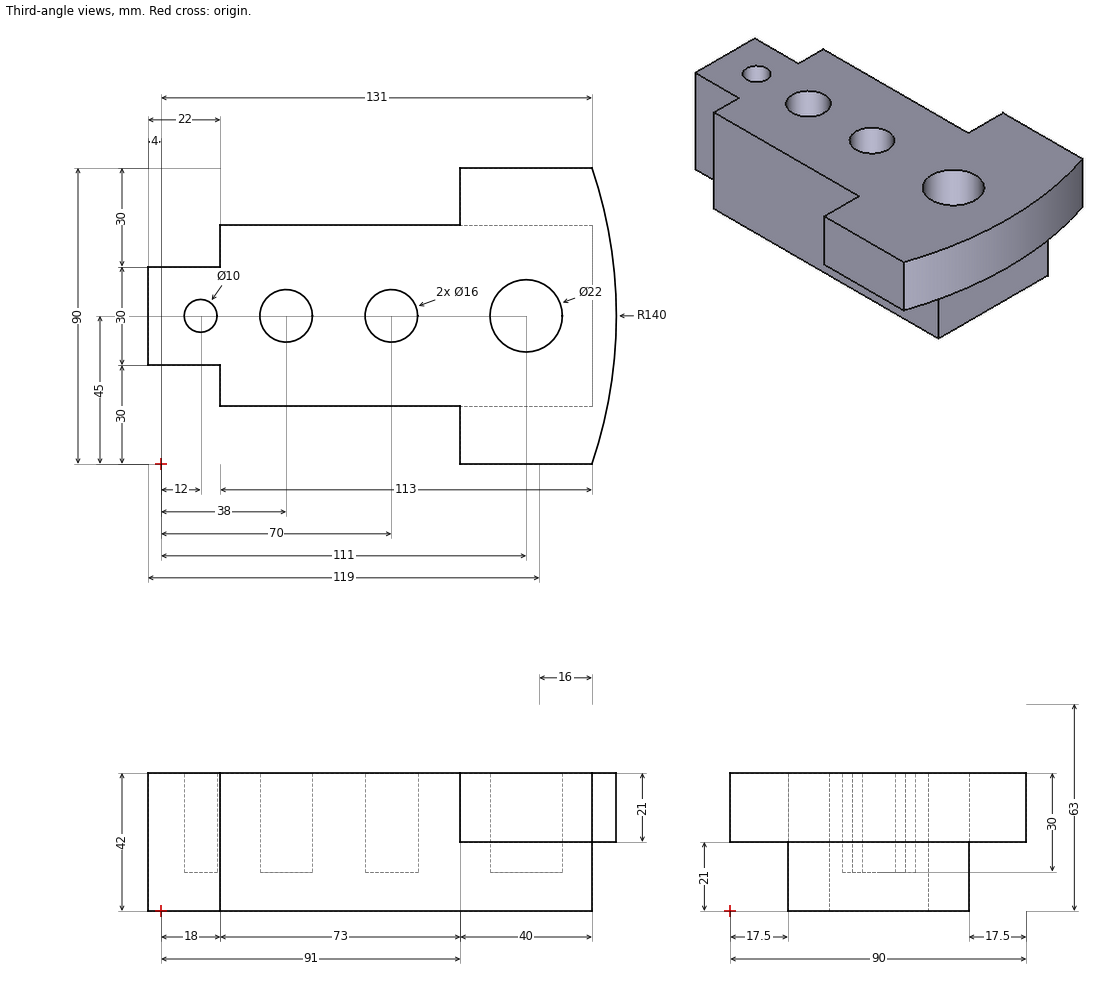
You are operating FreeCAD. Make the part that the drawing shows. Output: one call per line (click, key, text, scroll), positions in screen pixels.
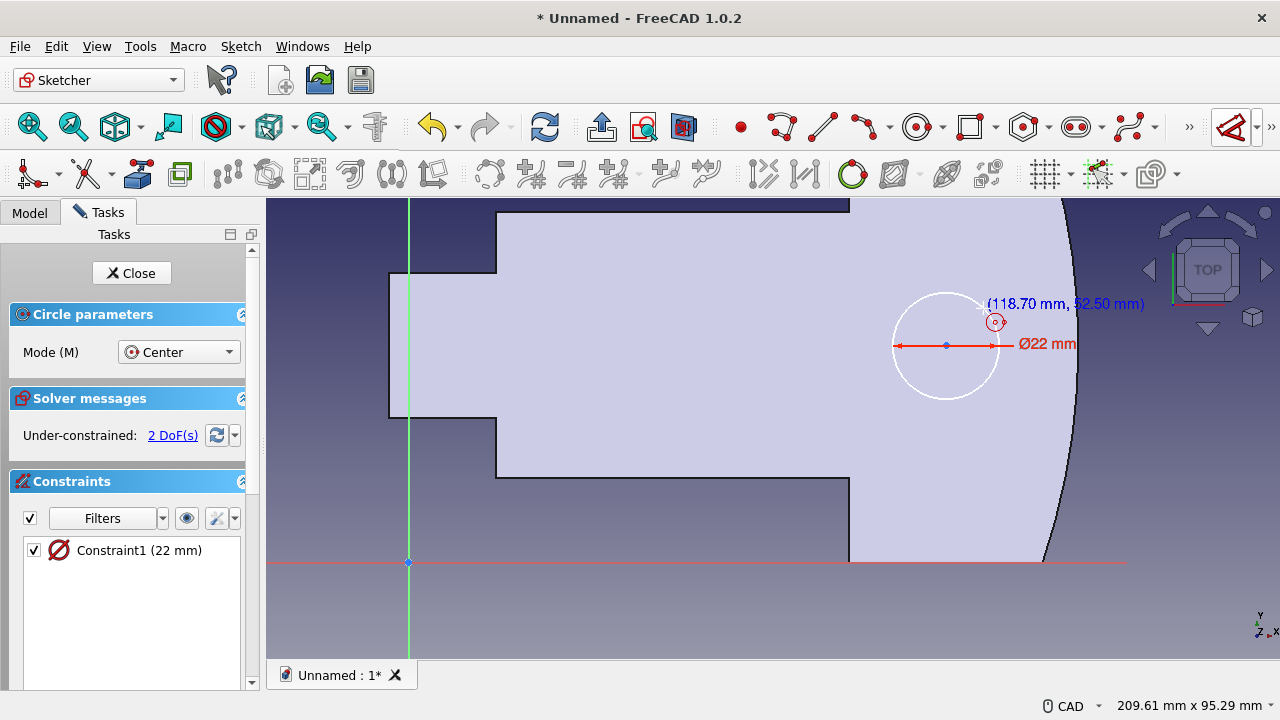
click(747, 345)
move(775, 318)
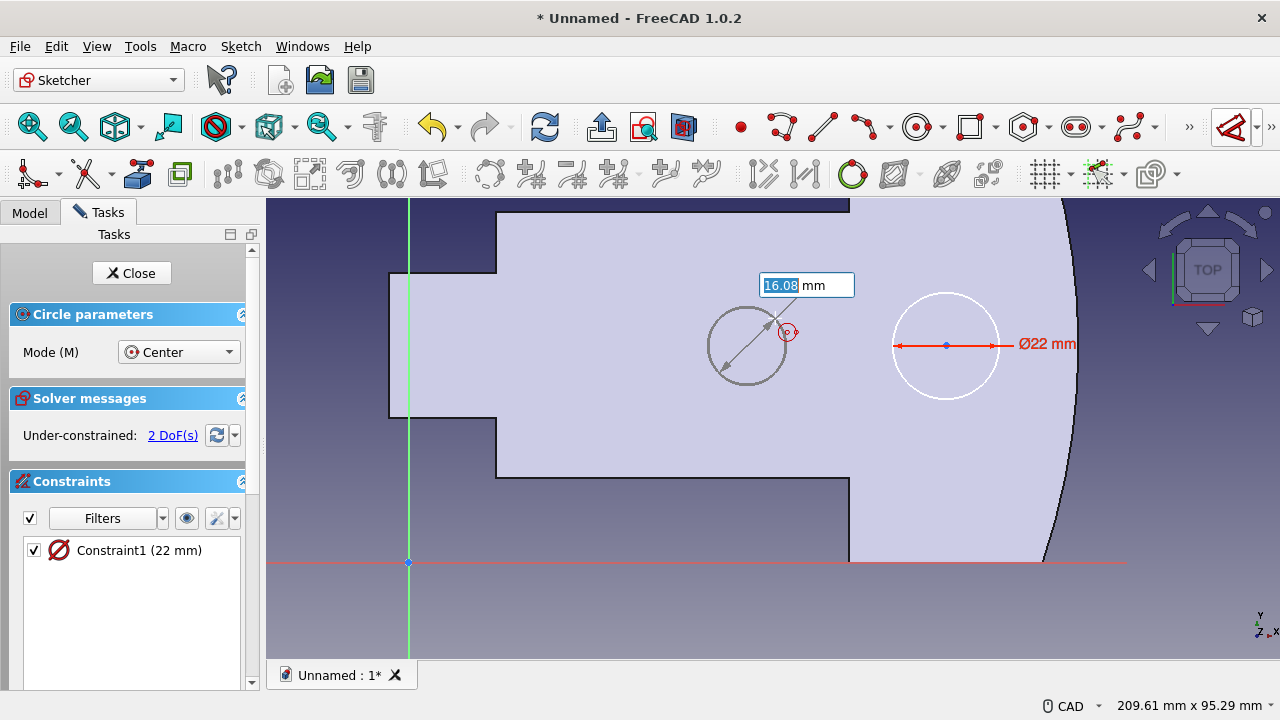
text(16)
key(Return)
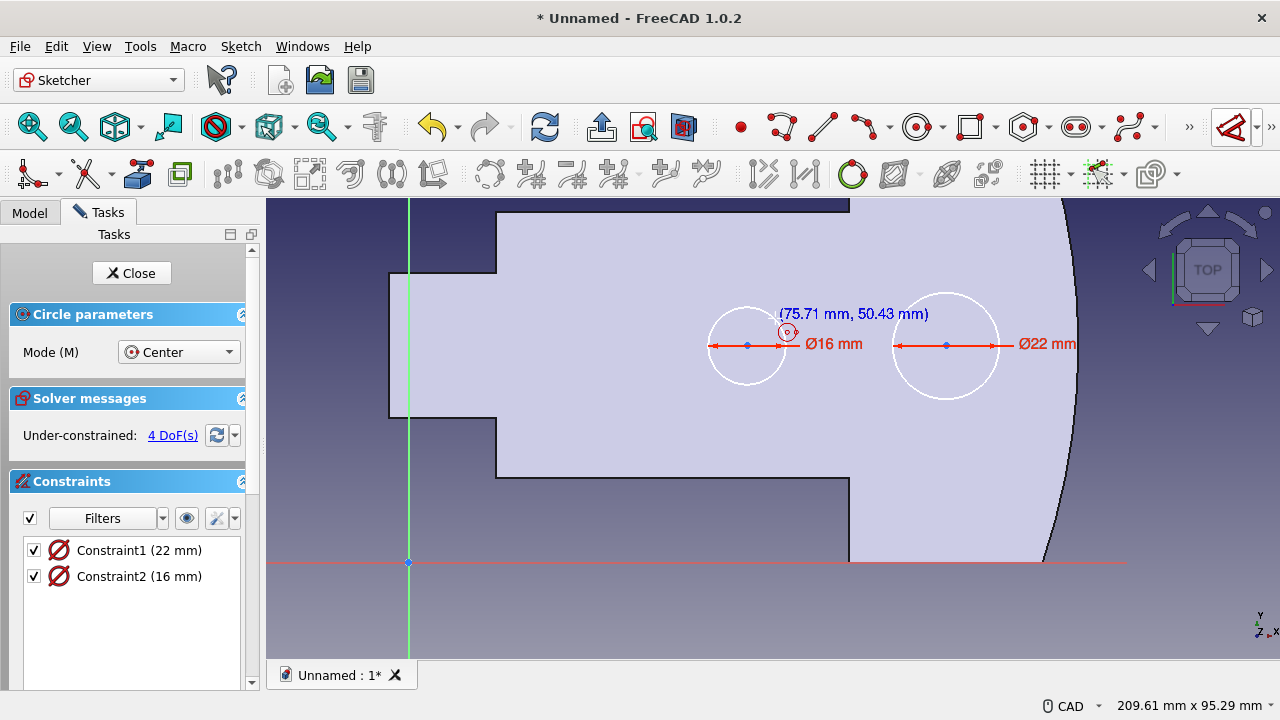
click(593, 345)
move(620, 318)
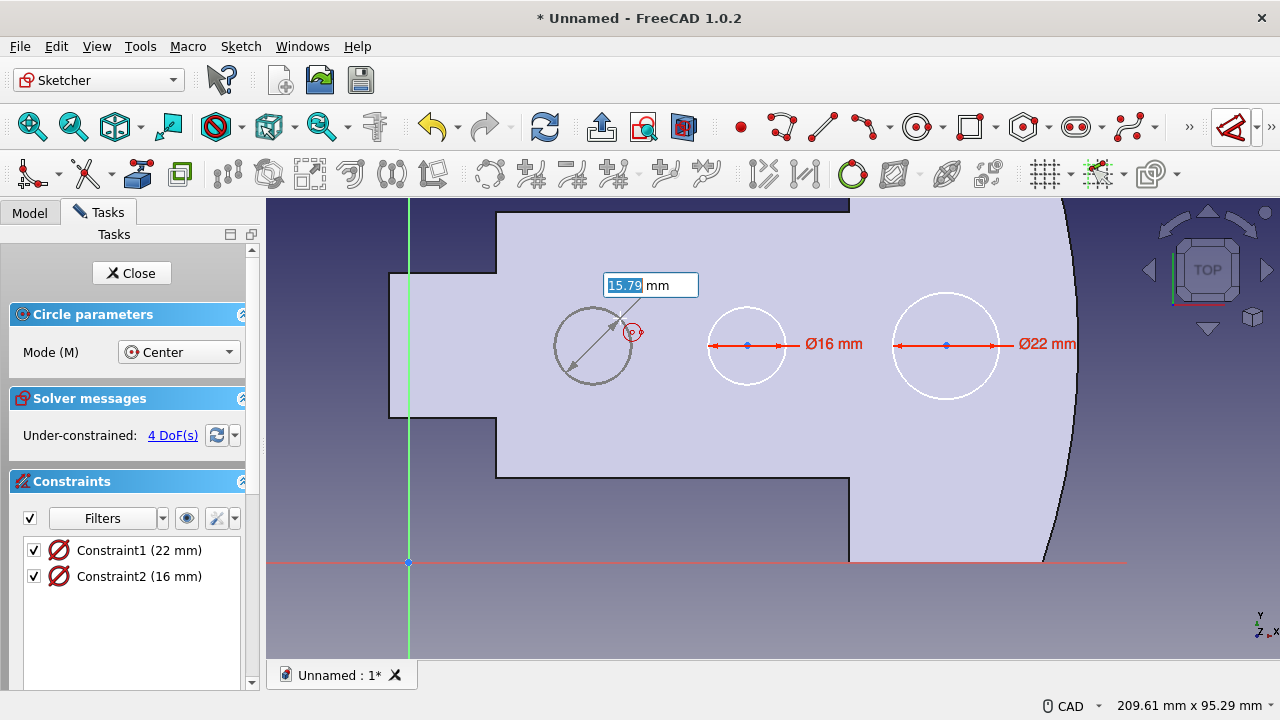
text(16)
key(Return)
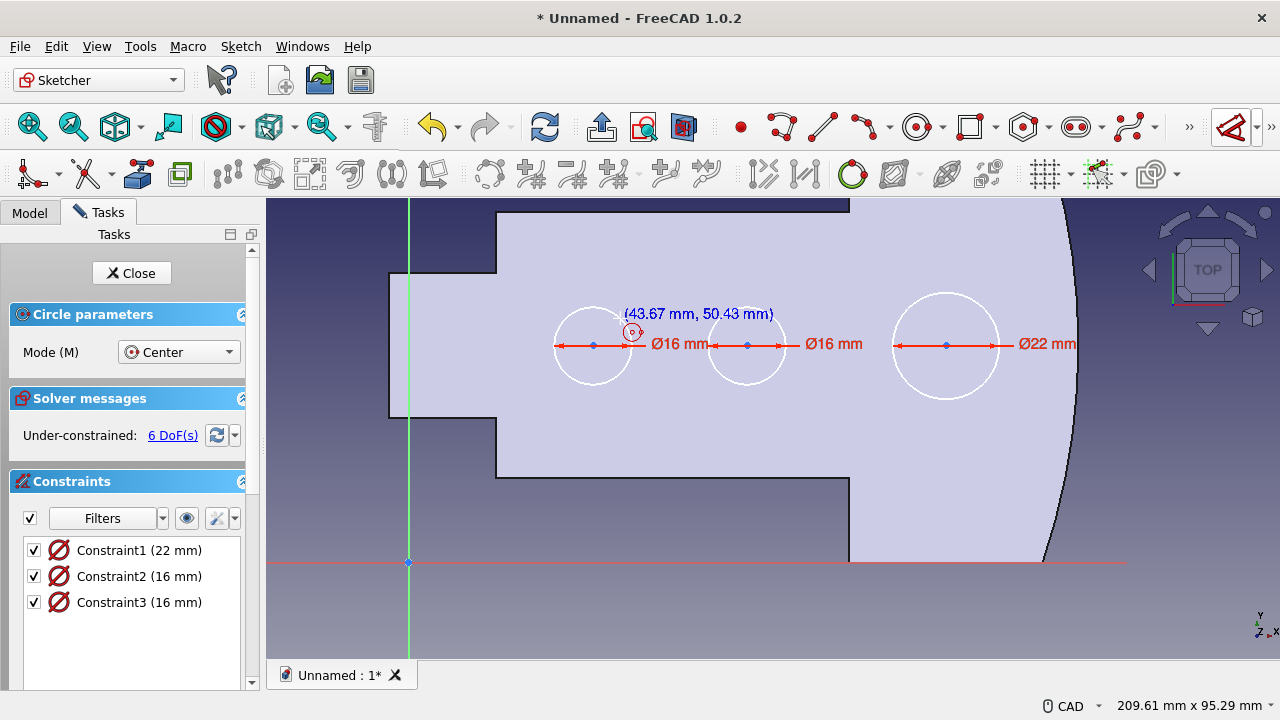
click(467, 345)
move(484, 328)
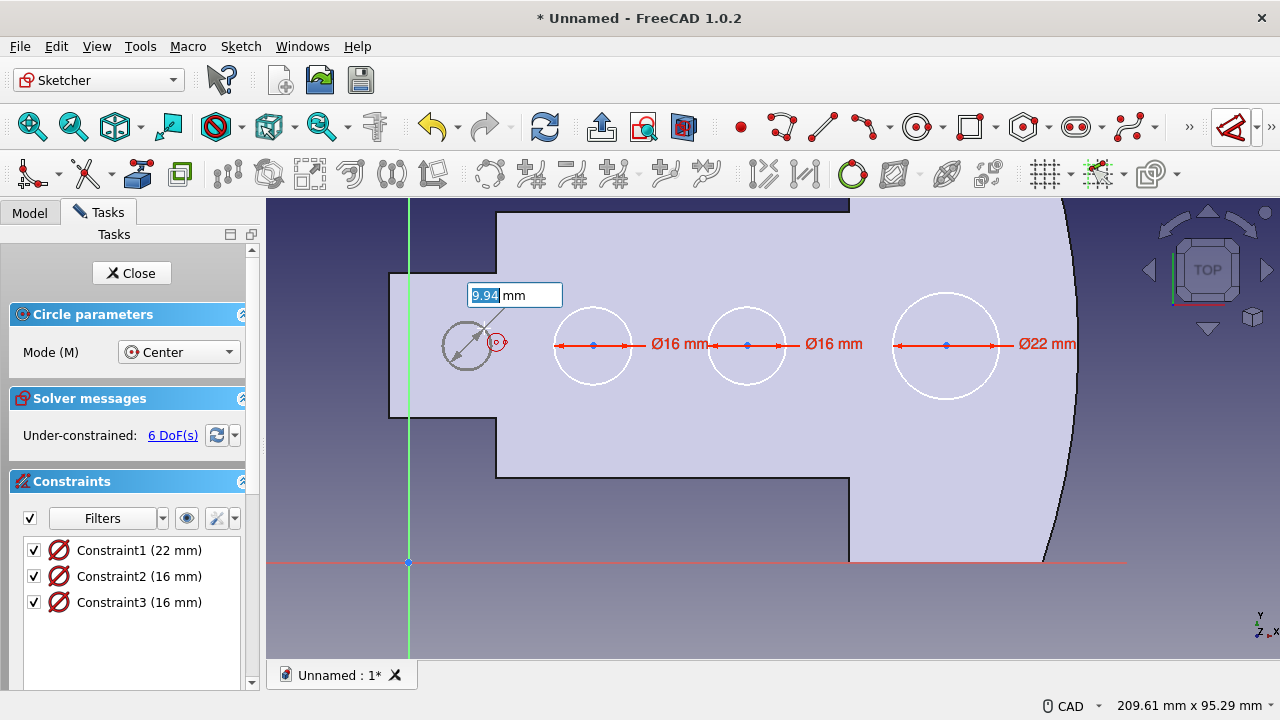
text(10)
key(Return)
key(Escape)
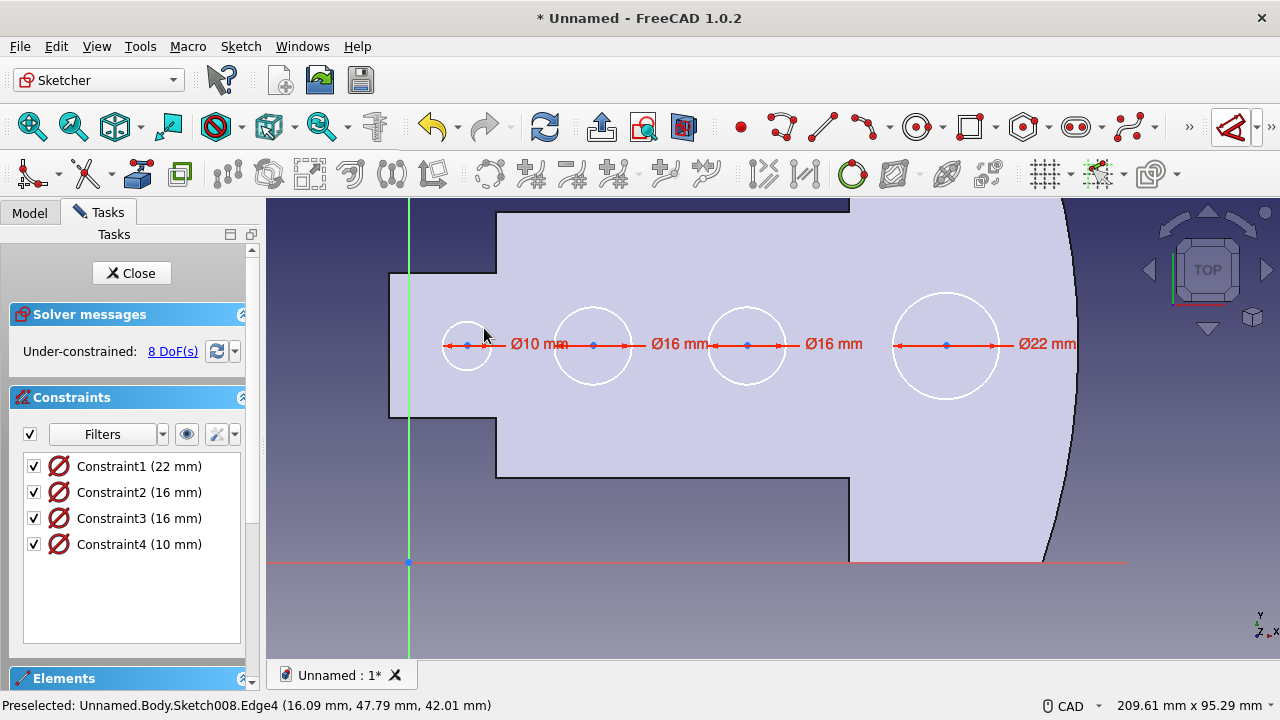
click(946, 346)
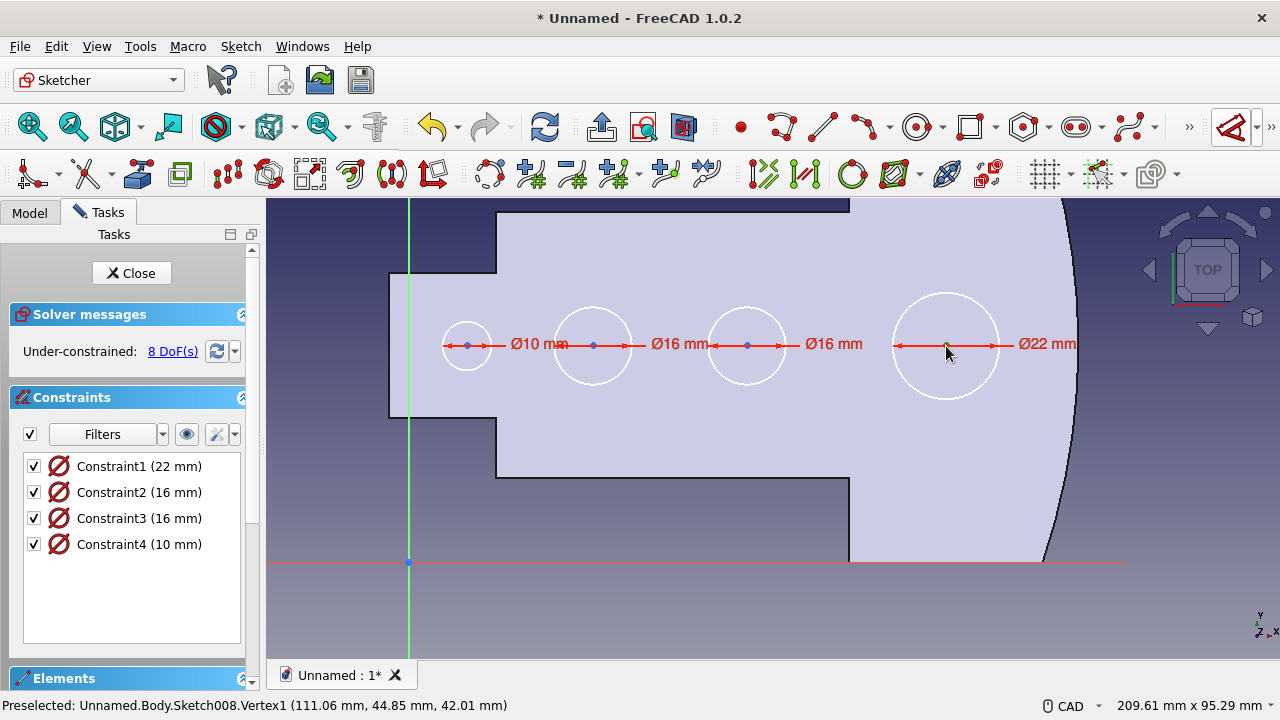
click(747, 346)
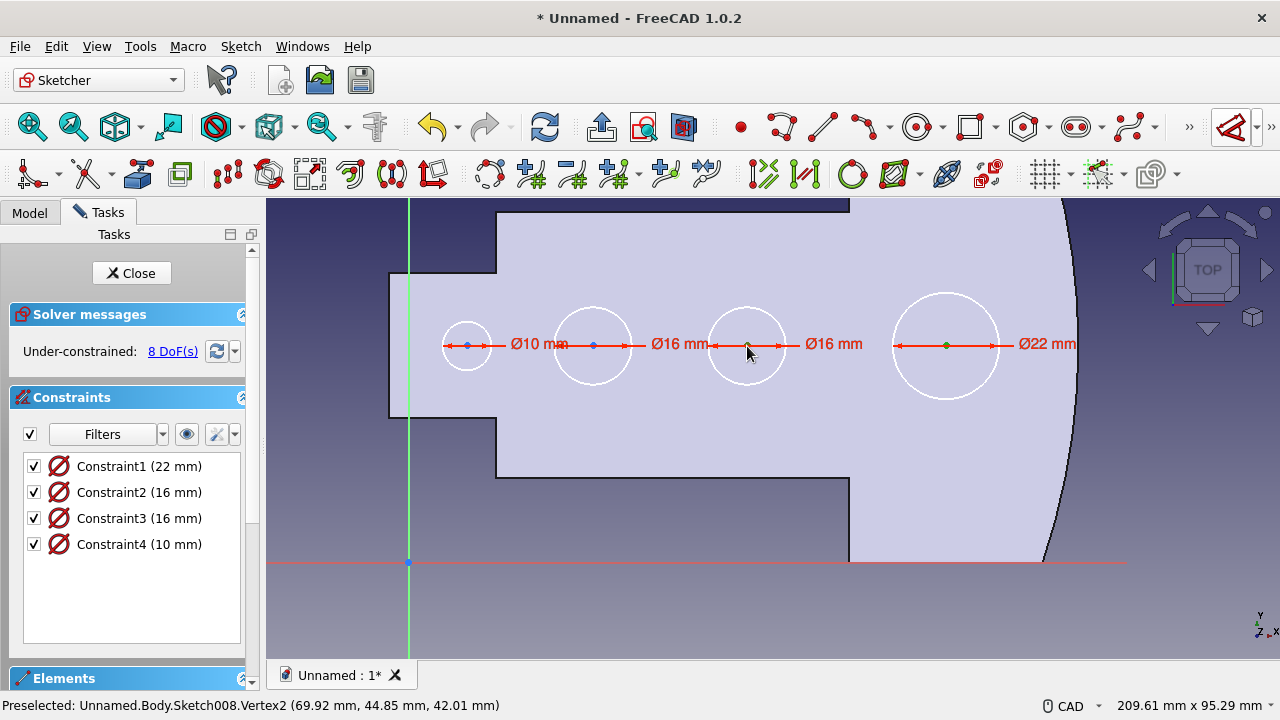
key(h)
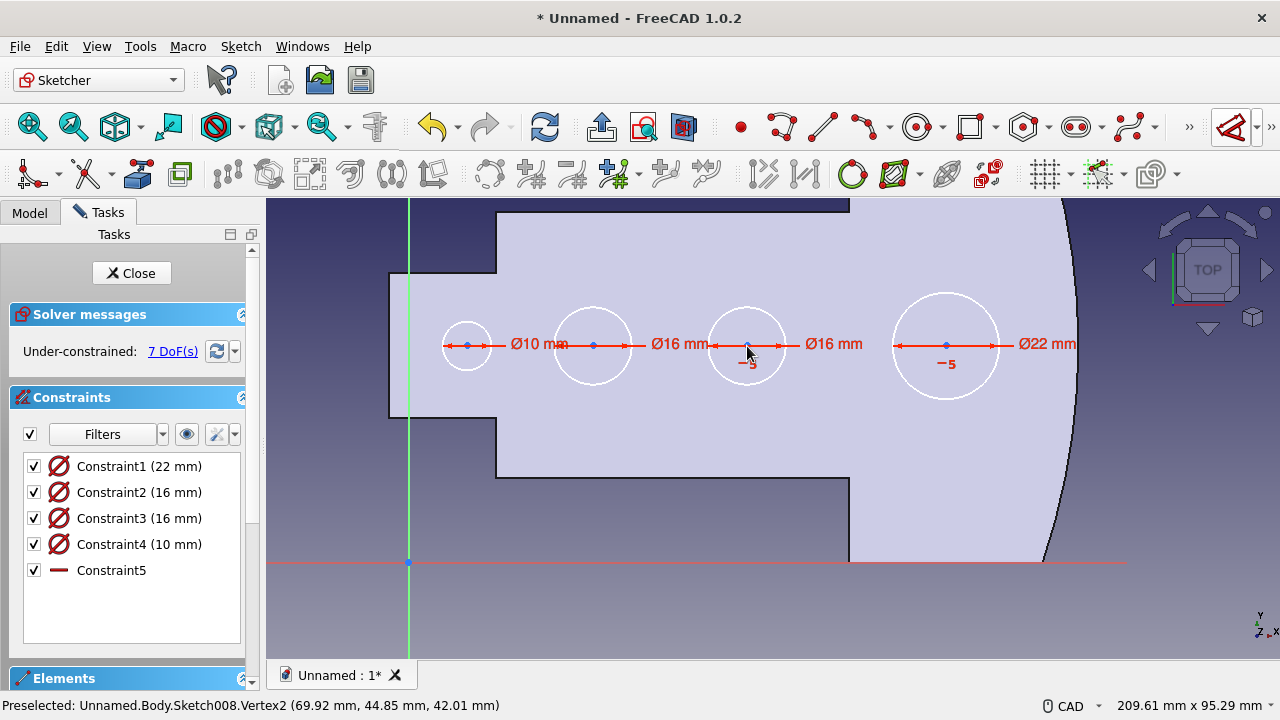
click(747, 346)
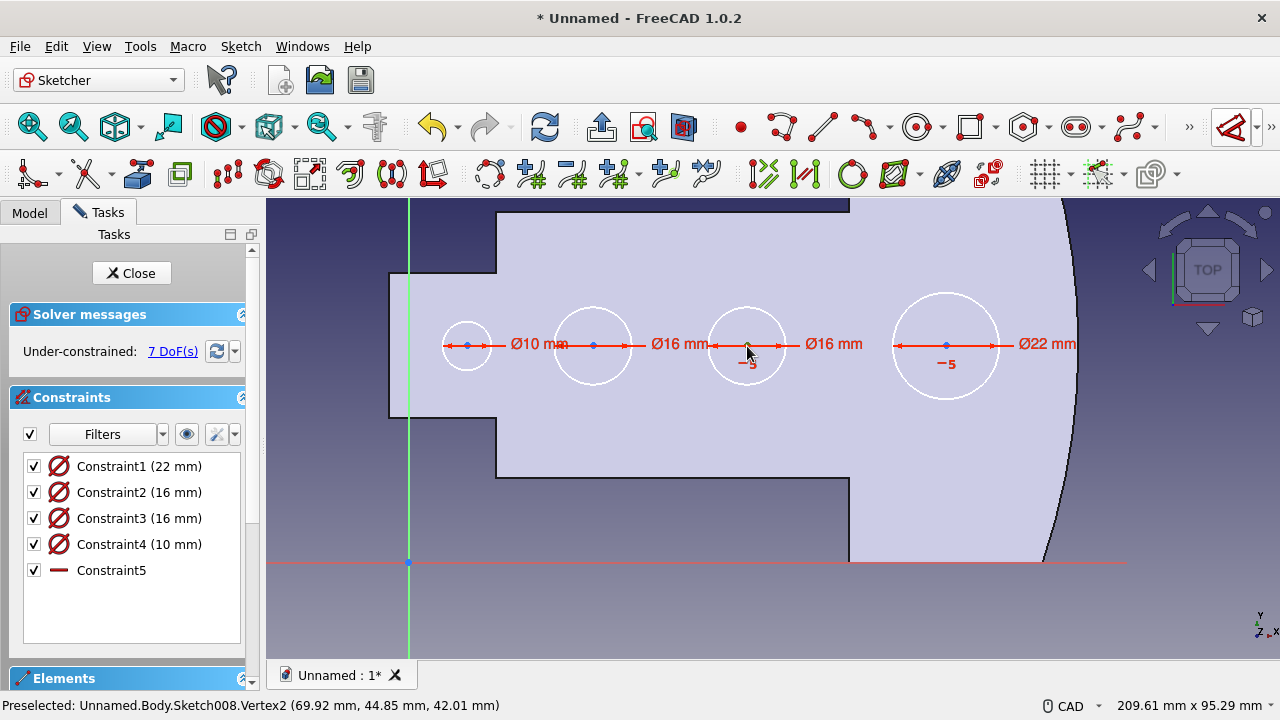
click(593, 346)